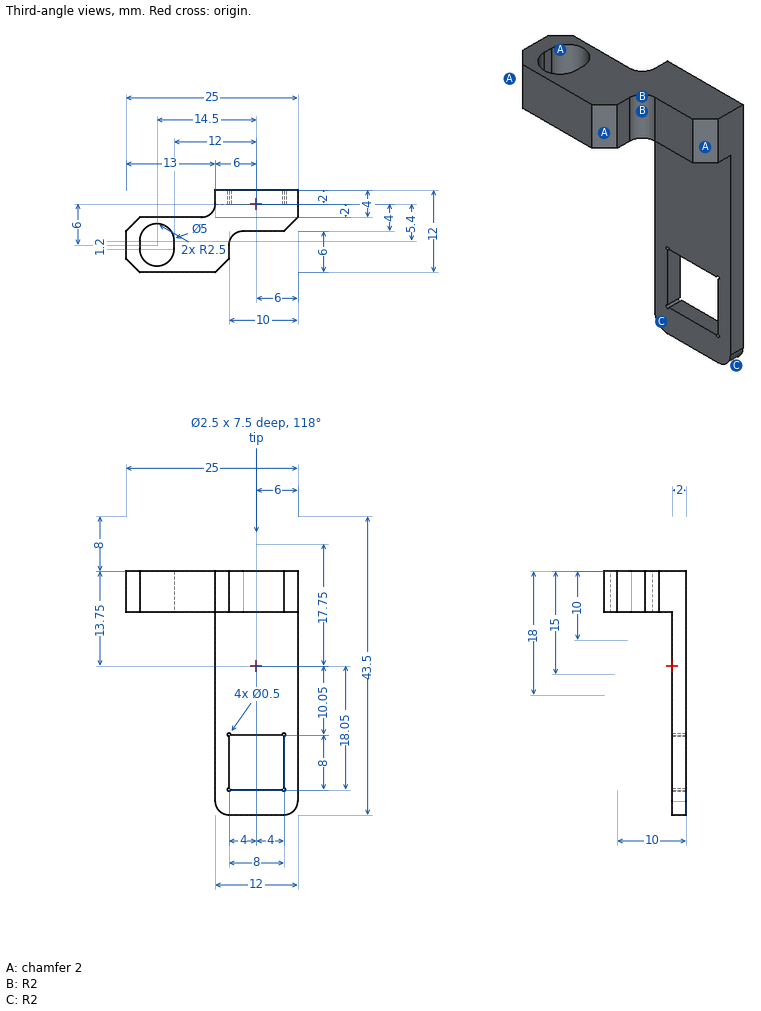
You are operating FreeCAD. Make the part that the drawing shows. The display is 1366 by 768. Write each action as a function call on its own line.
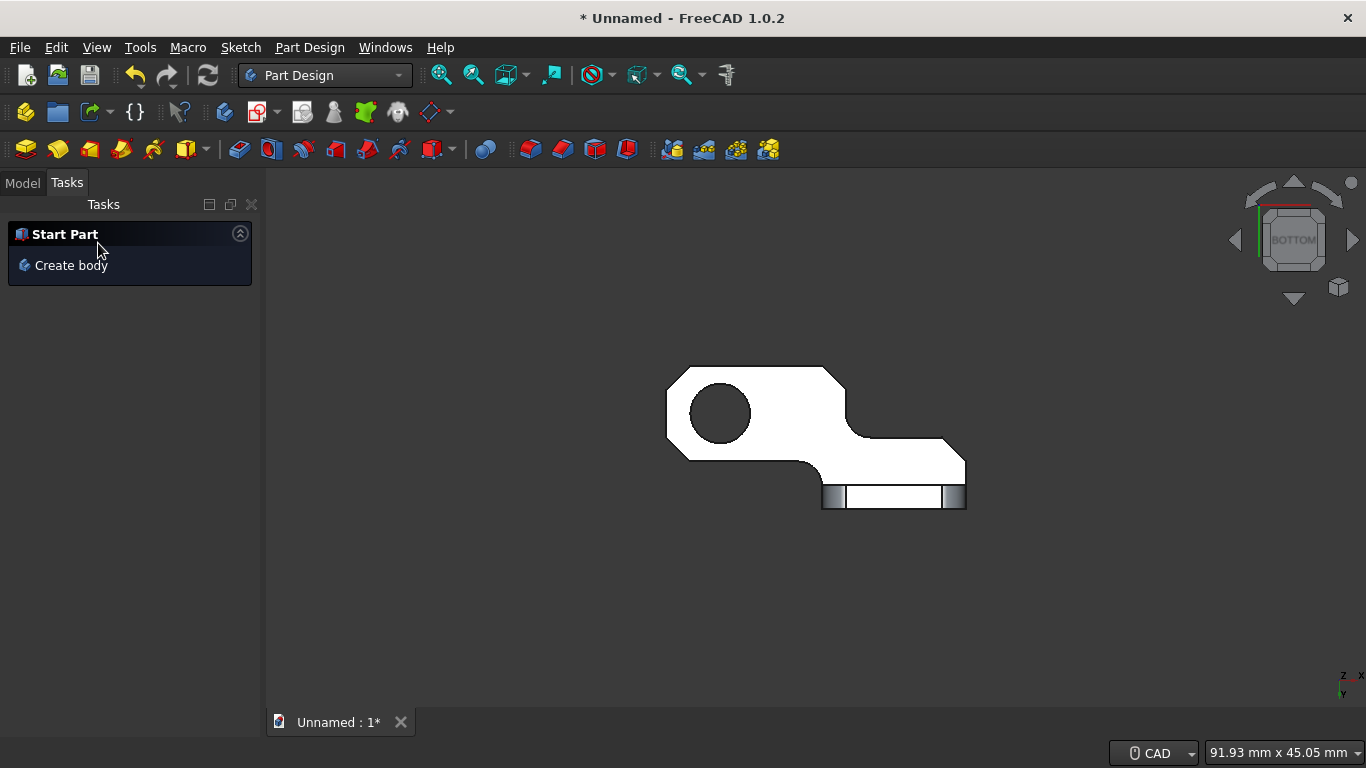
click(442, 76)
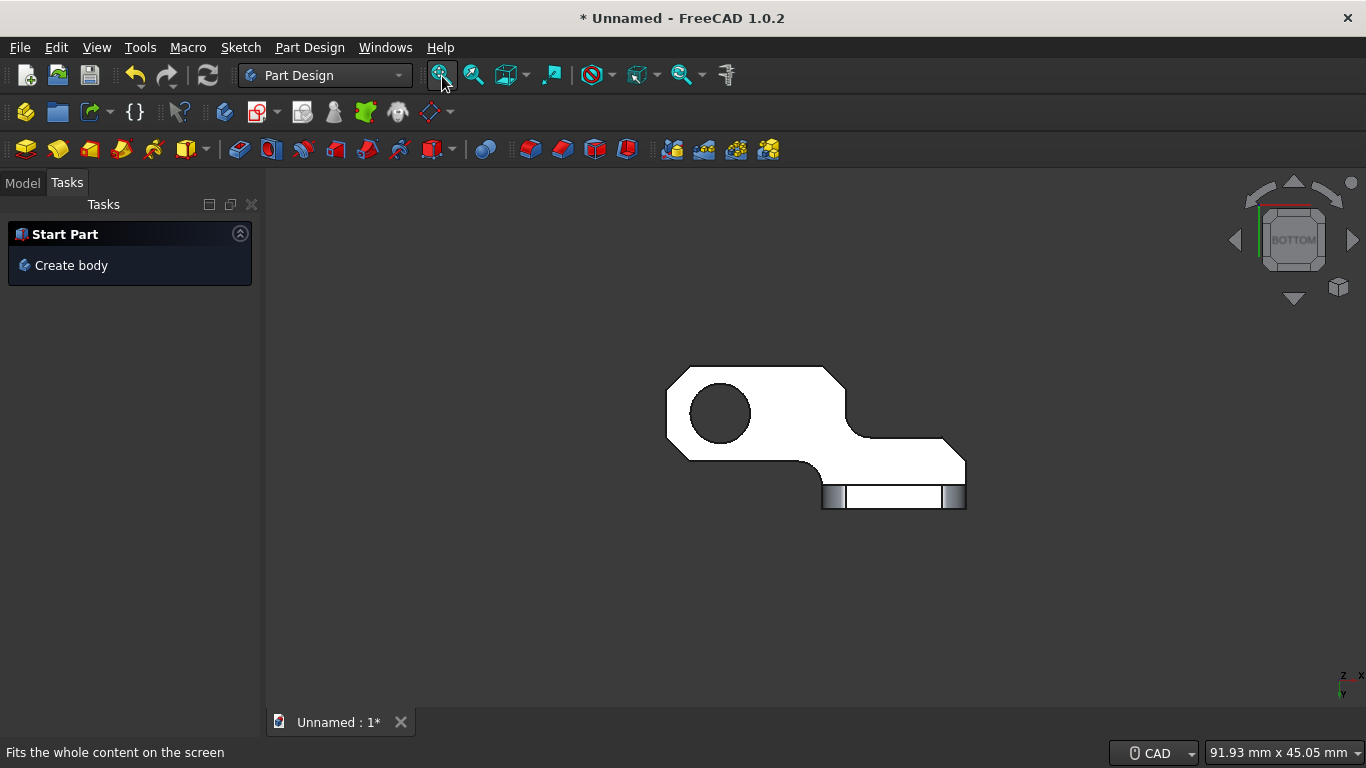
key(4)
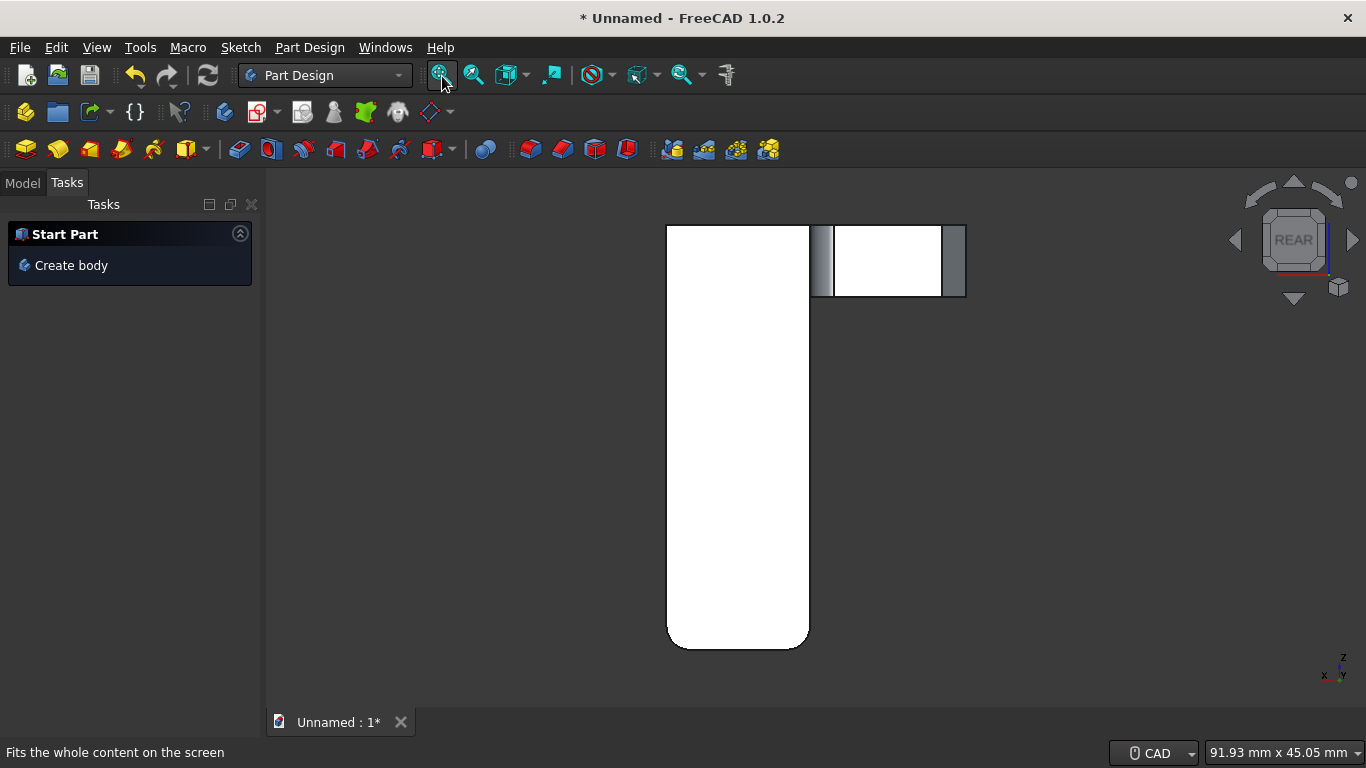
click(738, 315)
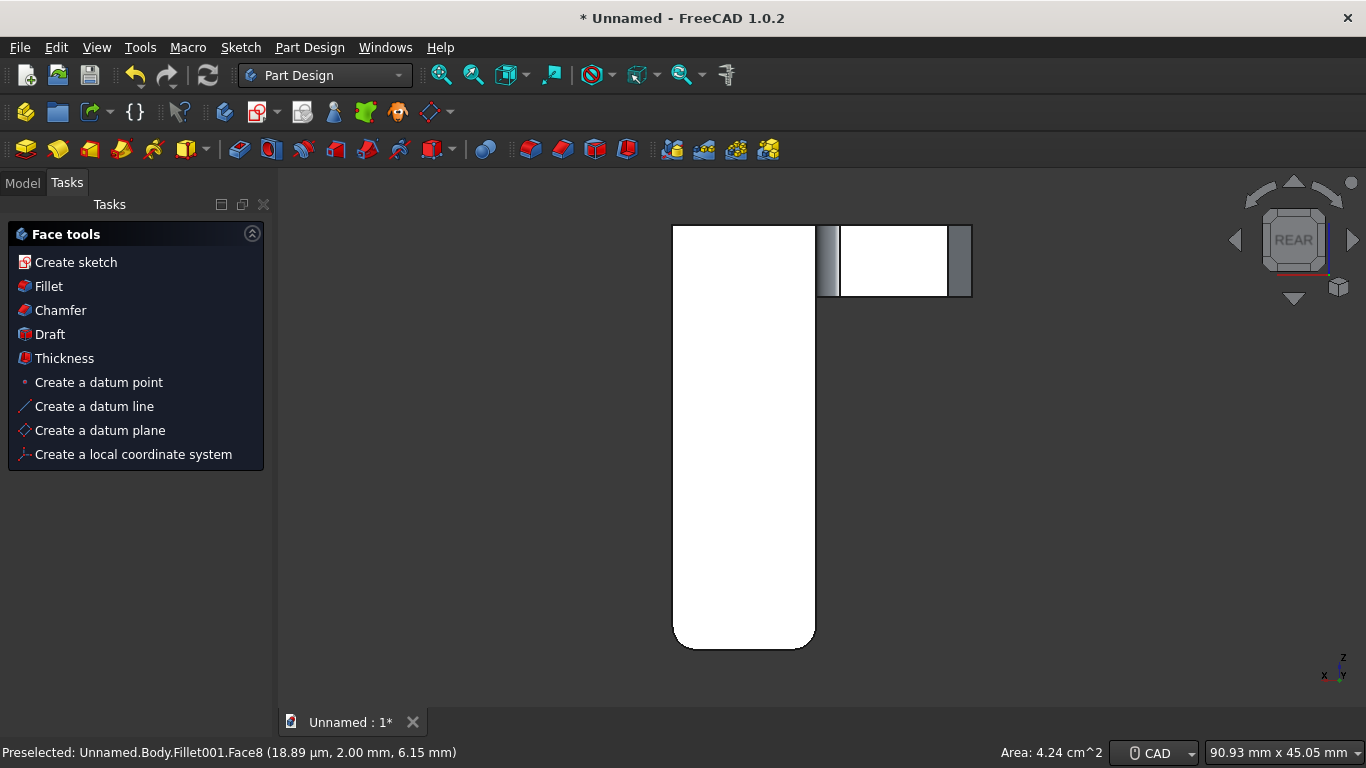
click(258, 112)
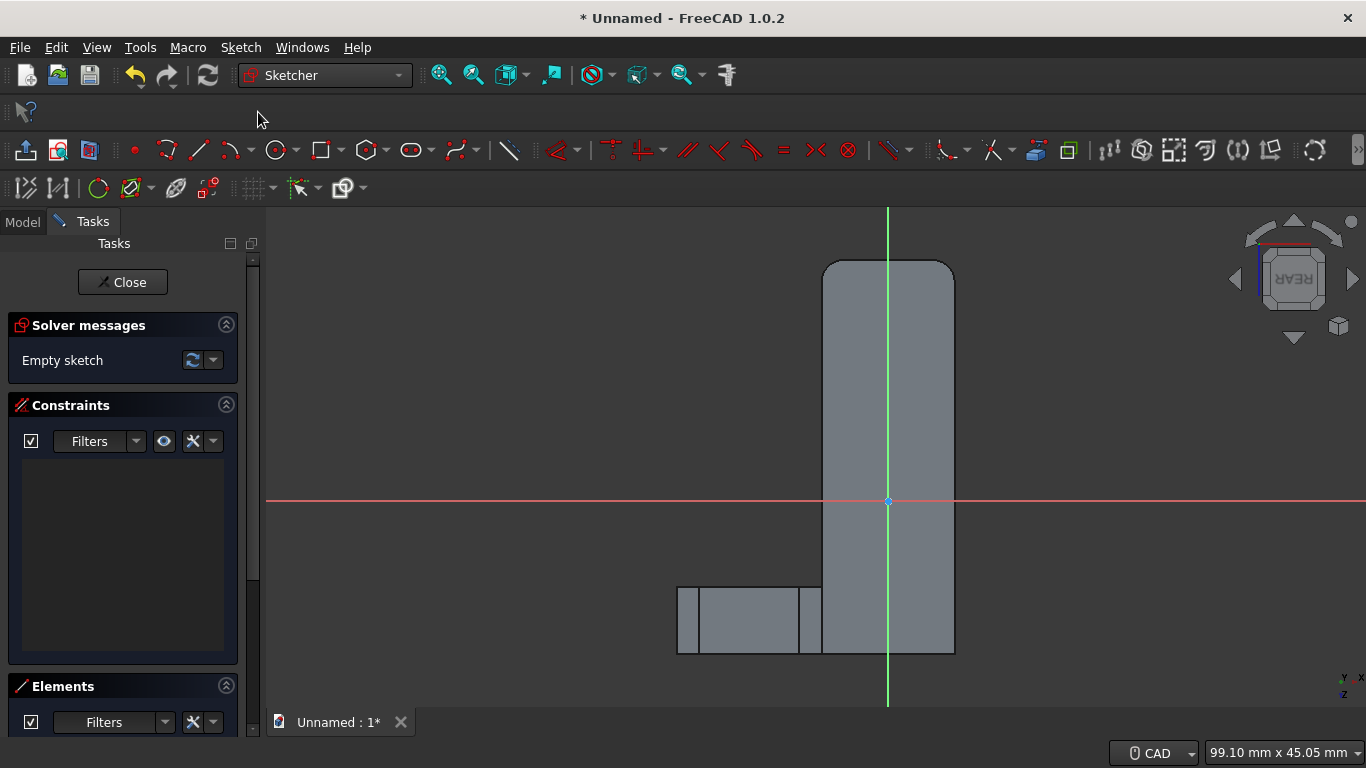
scroll(1174, 288, up, 2)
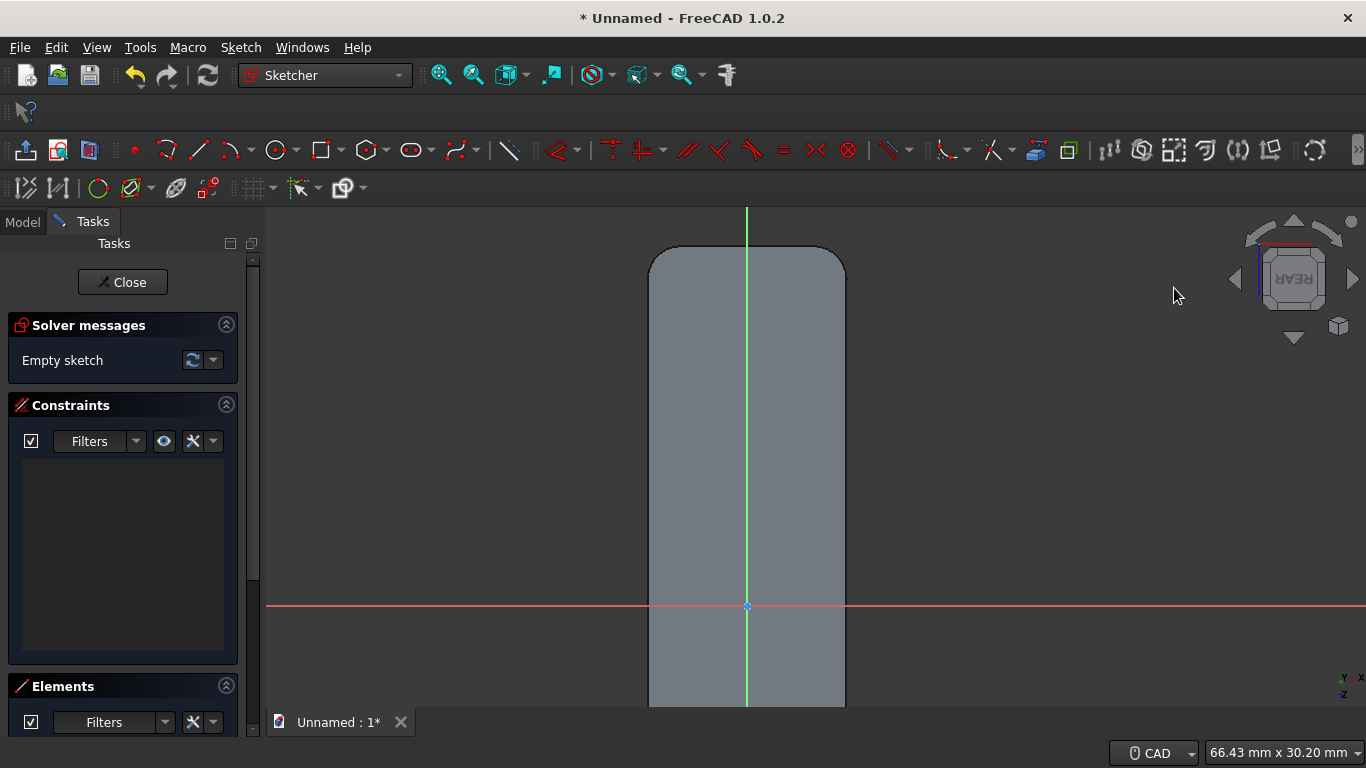
click(322, 150)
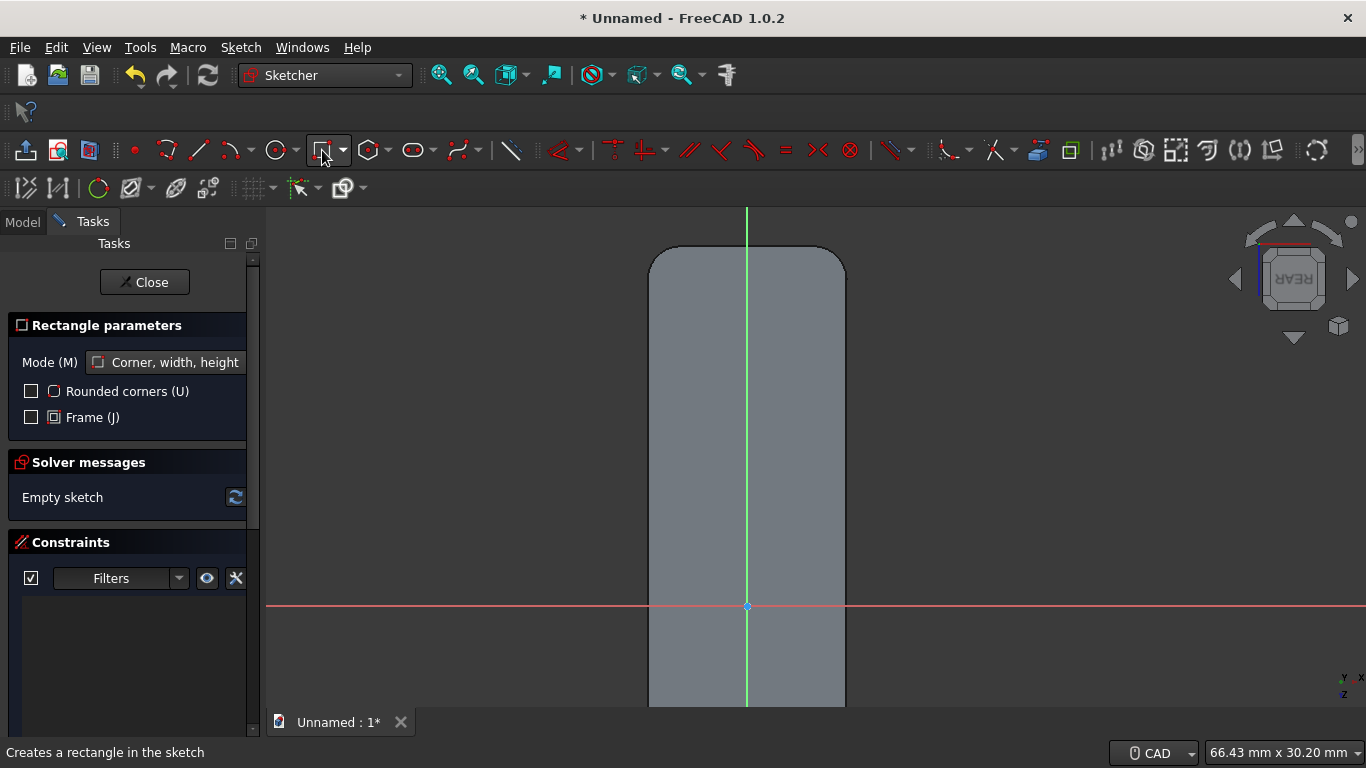
click(681, 307)
click(813, 440)
key(Escape)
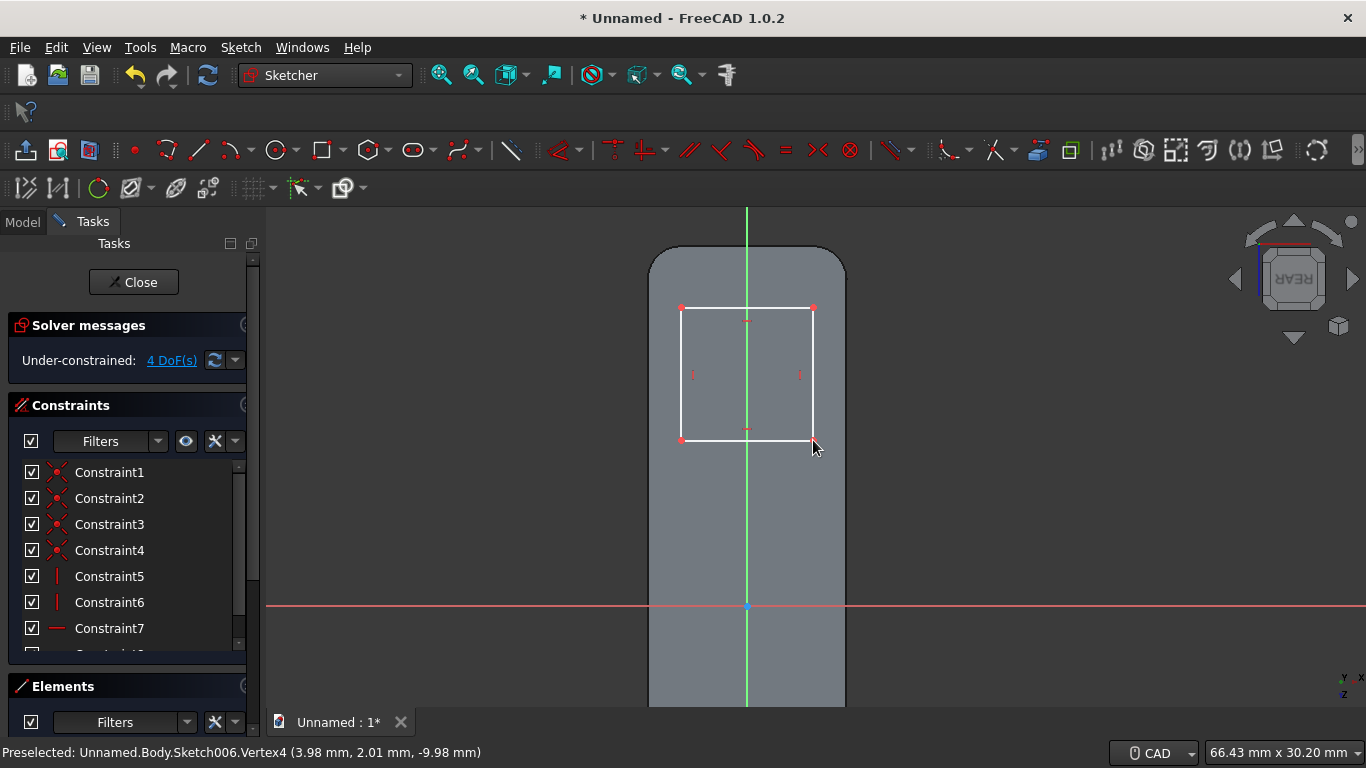
click(558, 150)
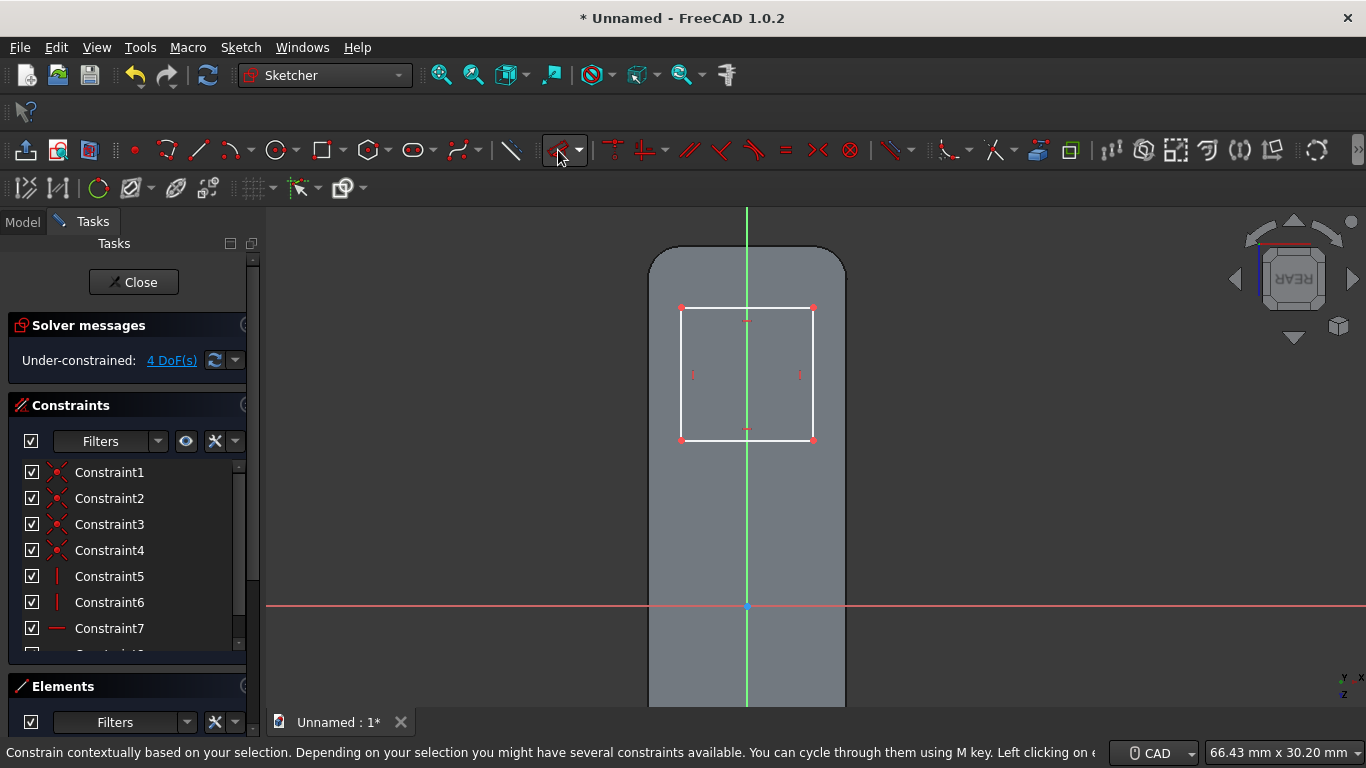
click(681, 348)
click(647, 375)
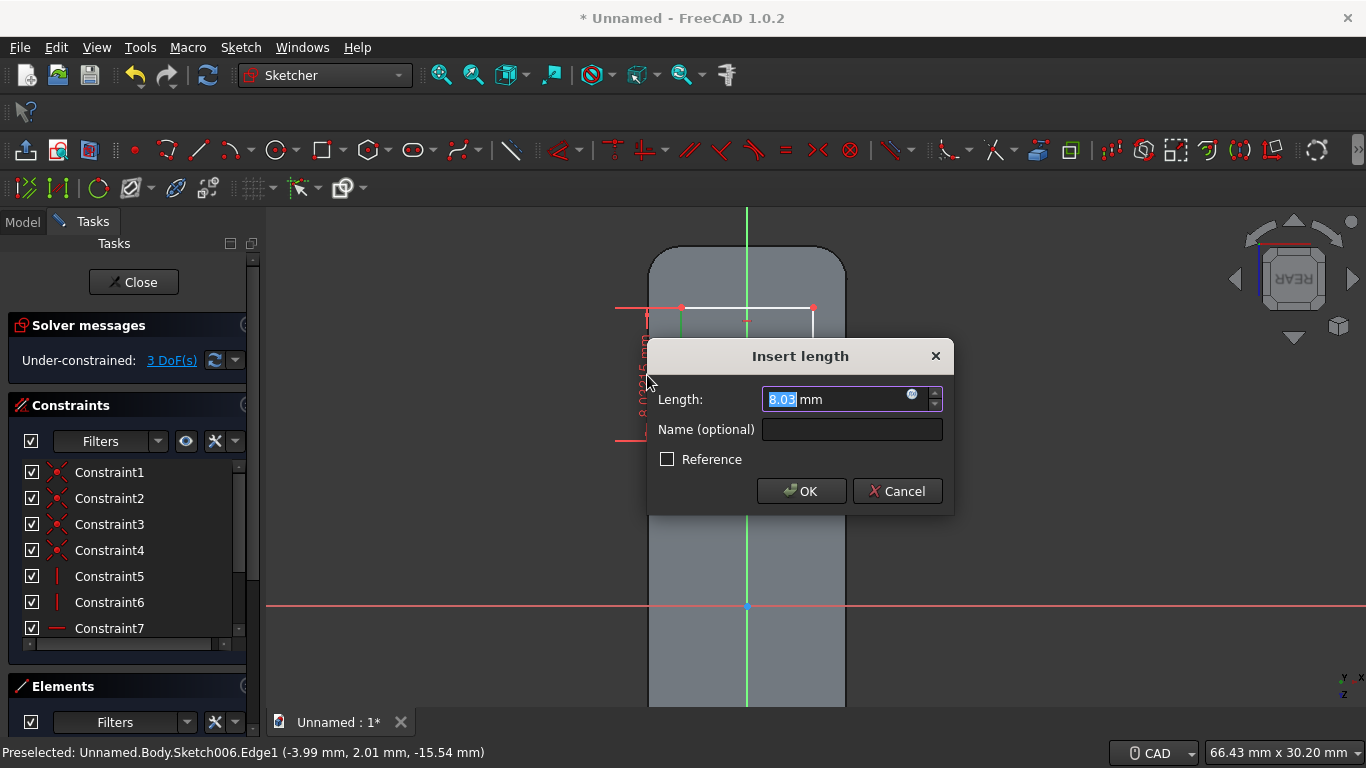
text(8)
key(Return)